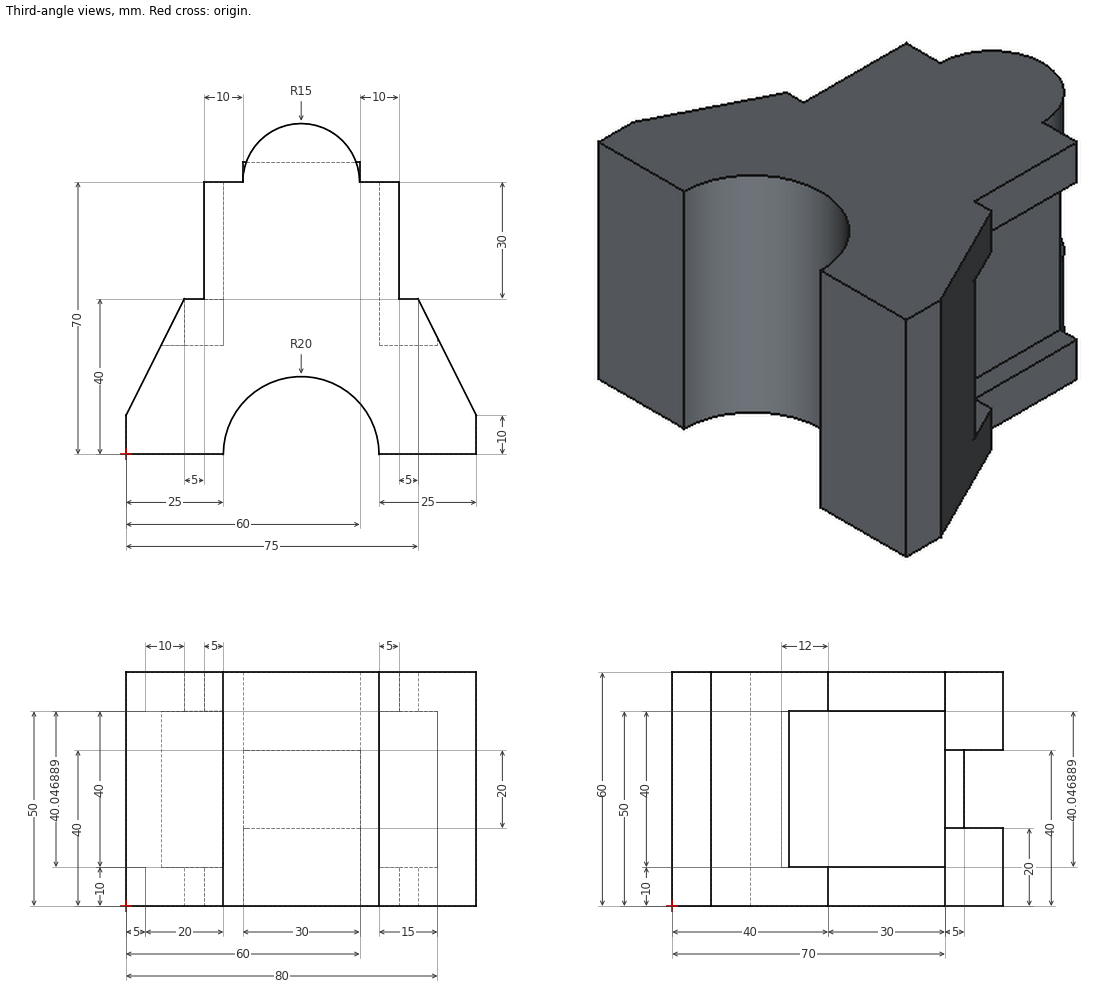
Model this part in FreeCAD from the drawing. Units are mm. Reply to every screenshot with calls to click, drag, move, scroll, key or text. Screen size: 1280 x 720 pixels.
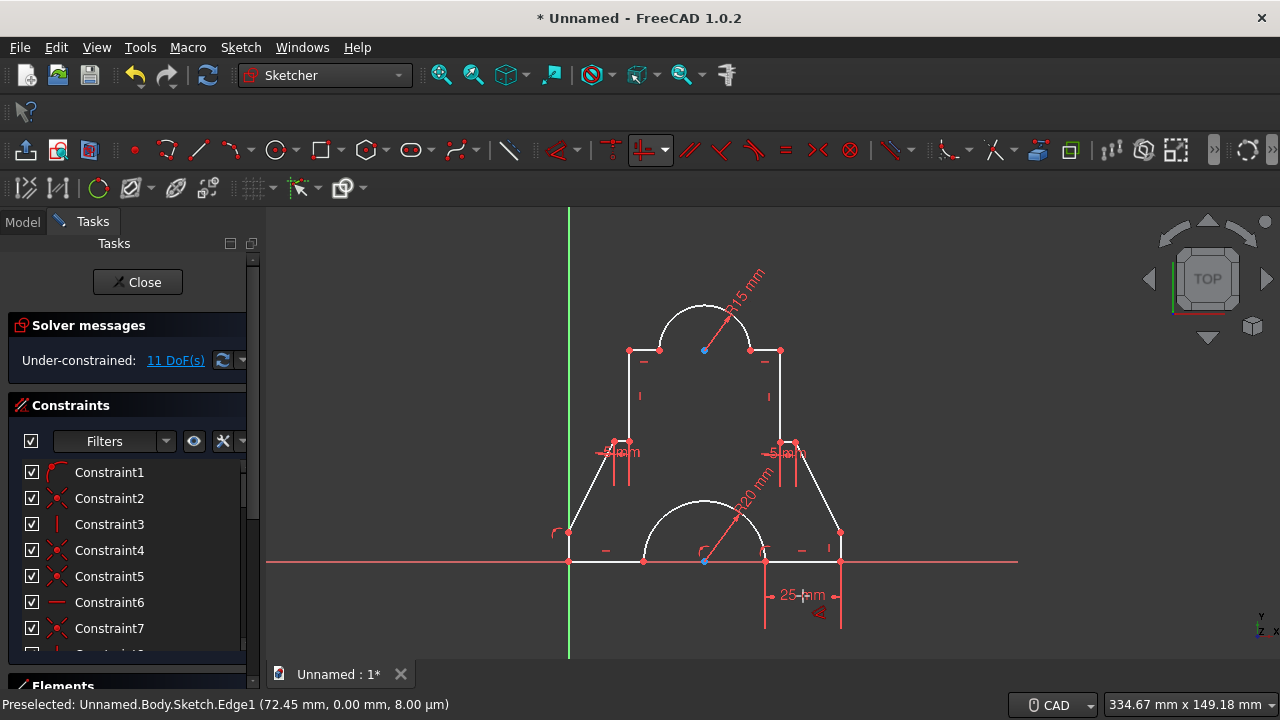
scroll(841, 550, up, 2)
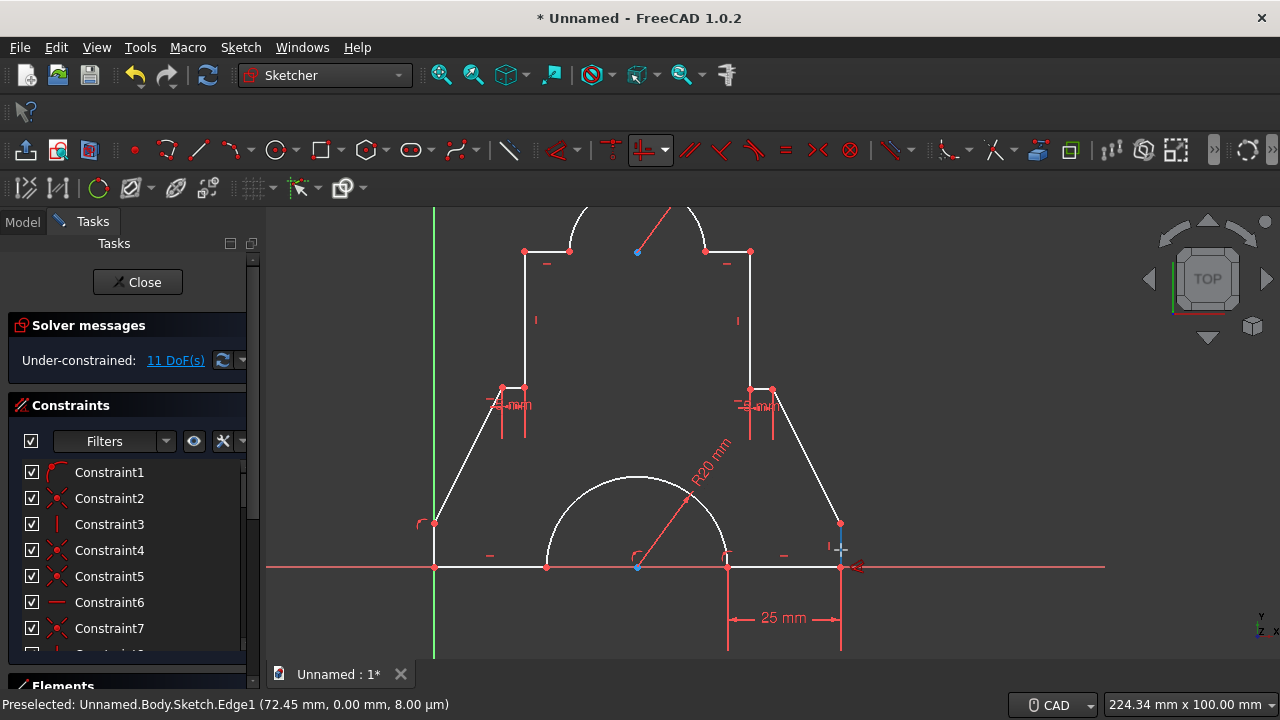
click(841, 550)
click(875, 546)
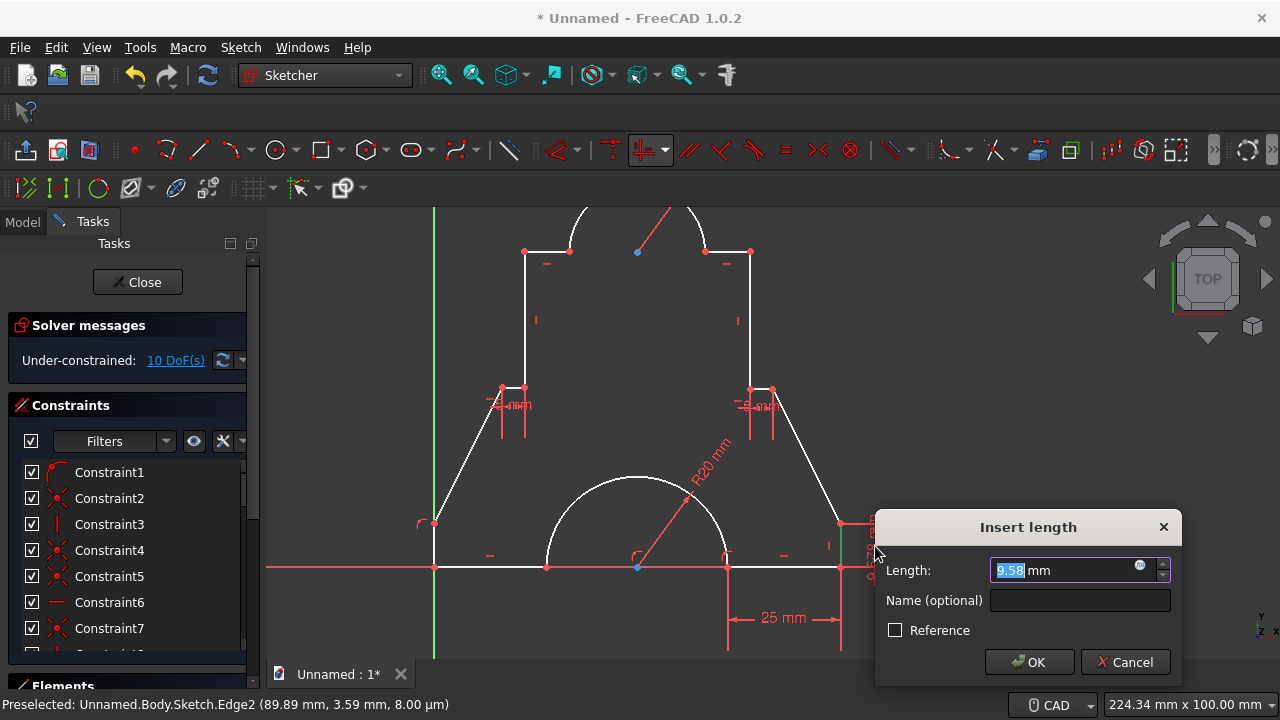
text(10)
key(Return)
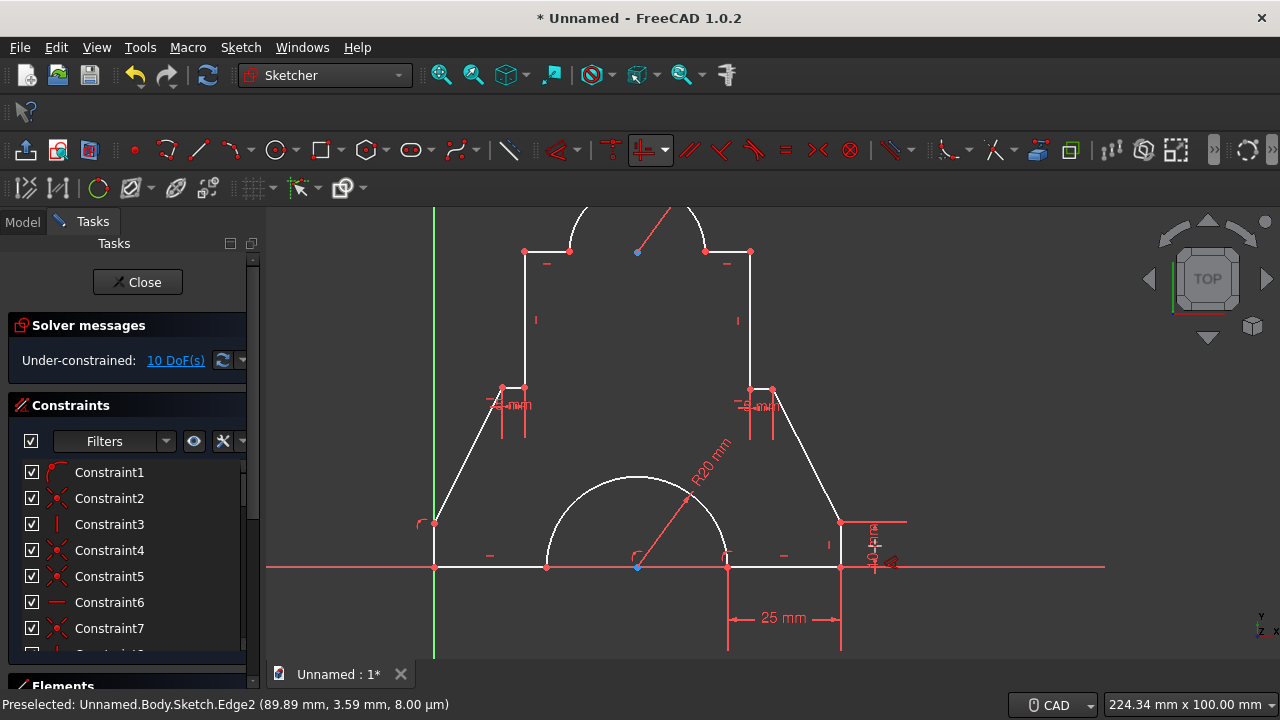
click(750, 348)
click(784, 321)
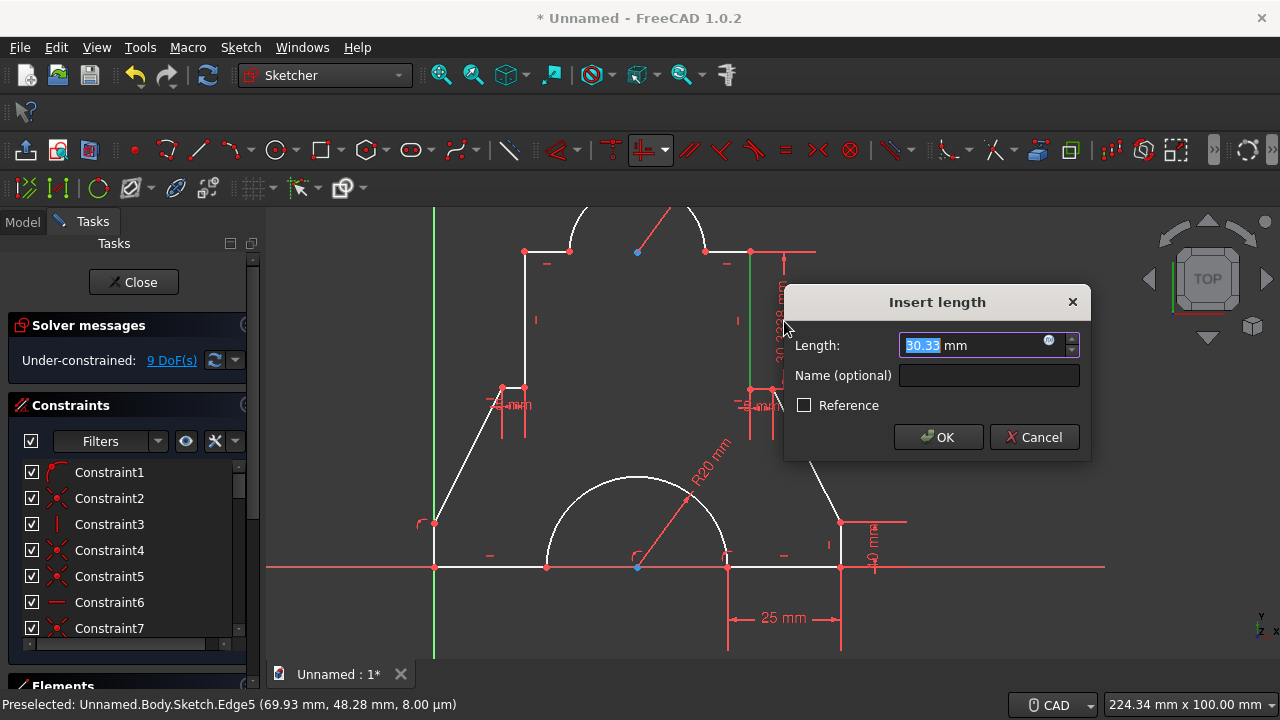
text(30)
key(Return)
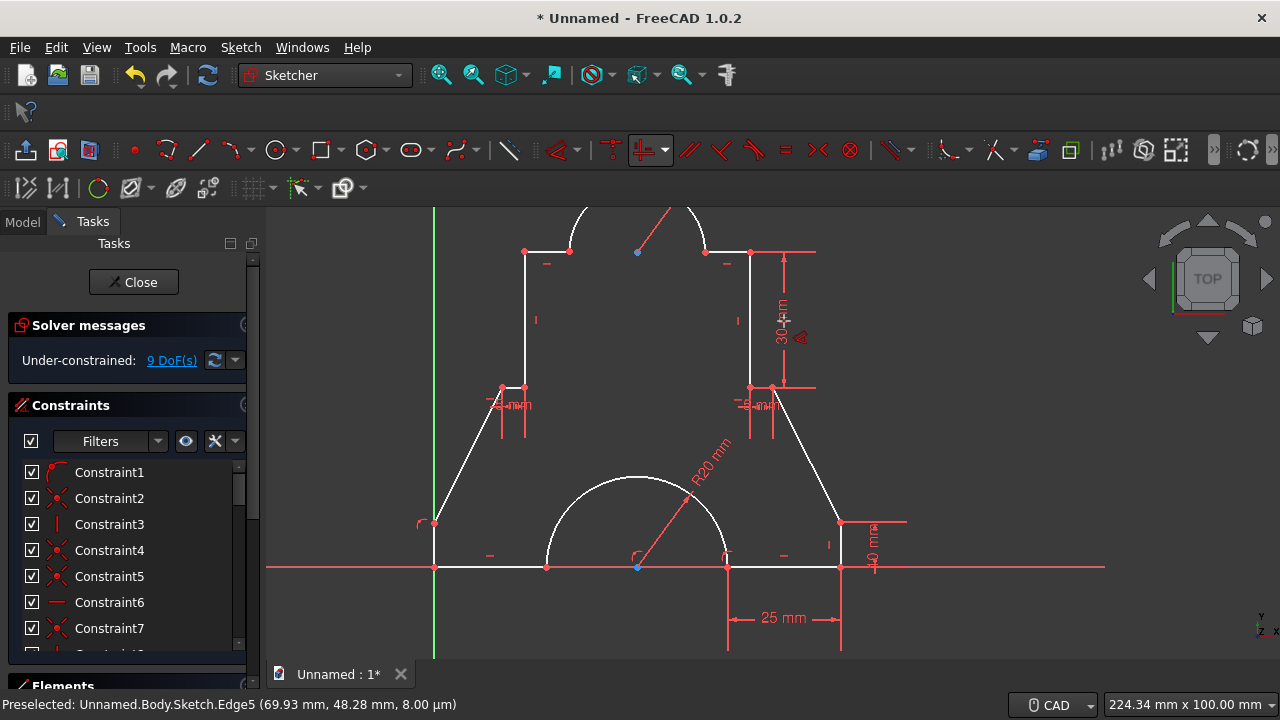
click(737, 252)
click(728, 286)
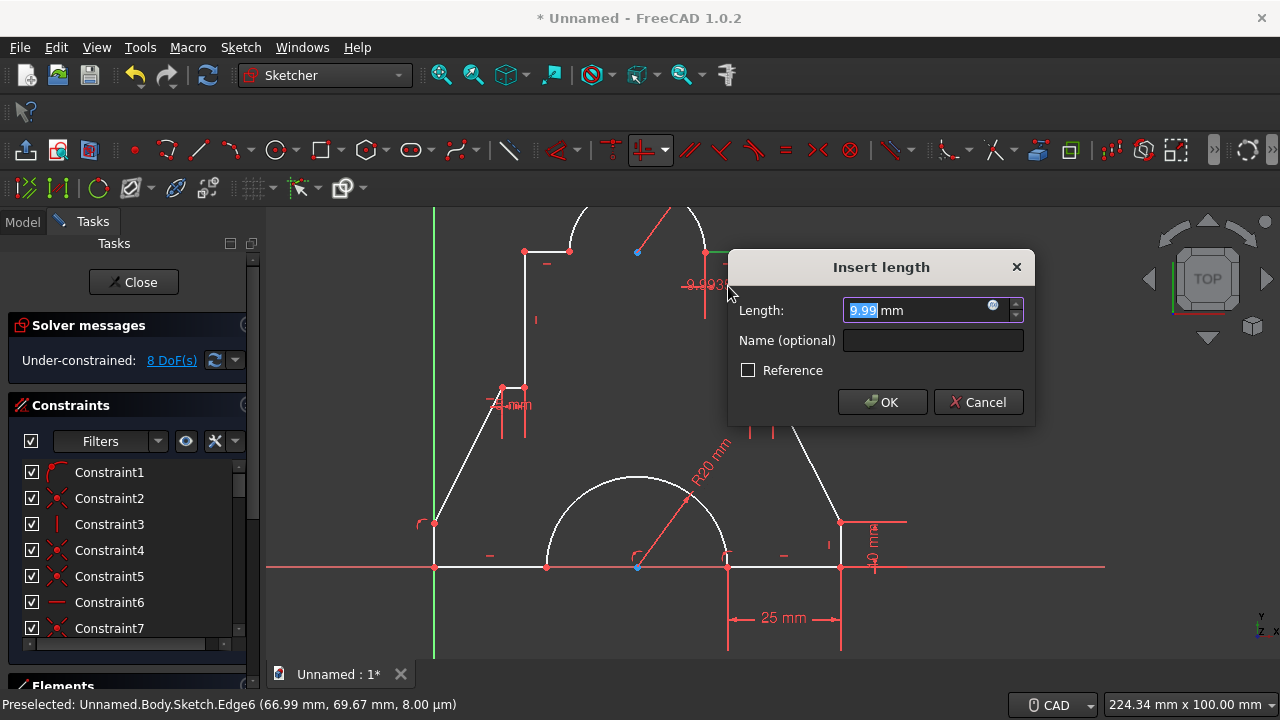
text(10)
key(Return)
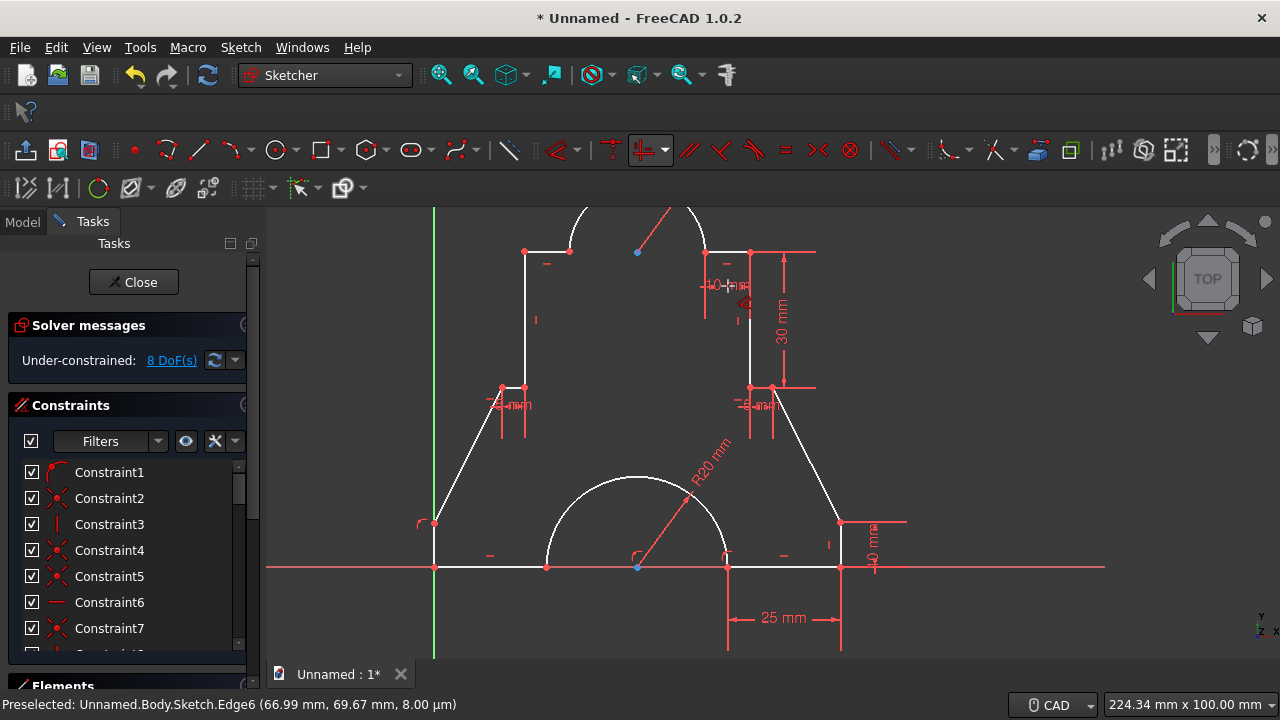
click(556, 252)
click(547, 286)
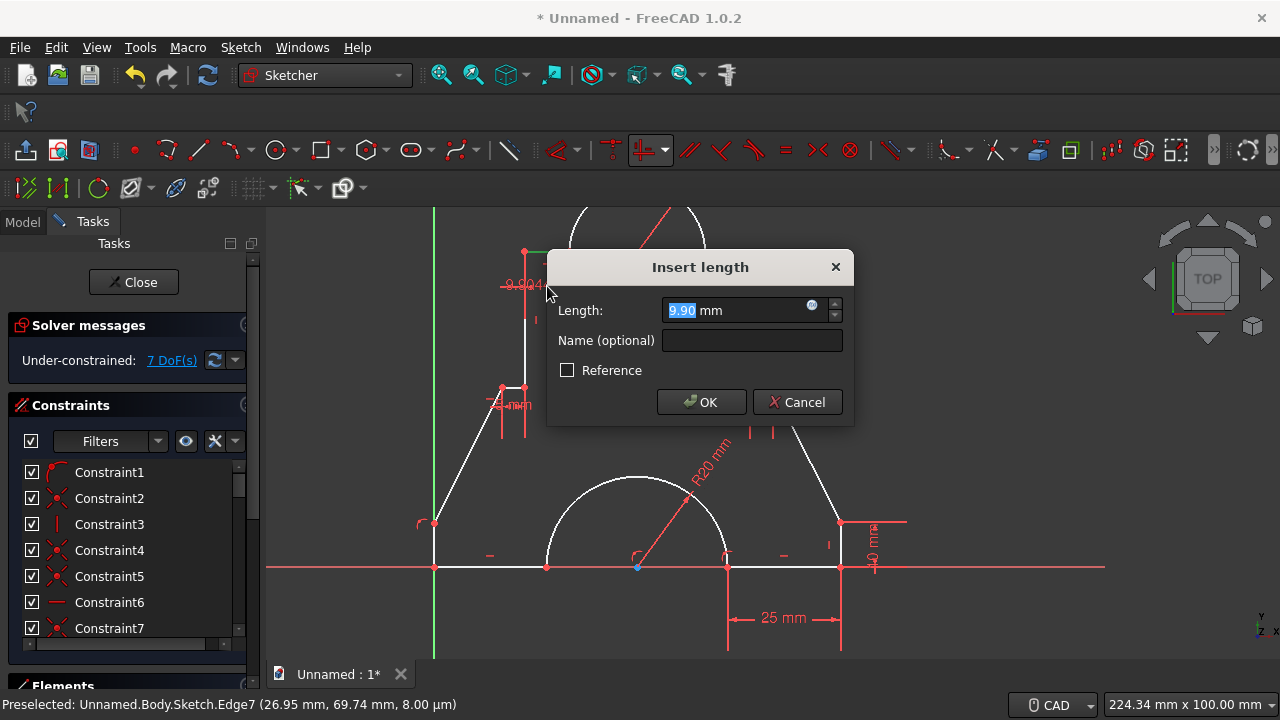
text(10)
key(Return)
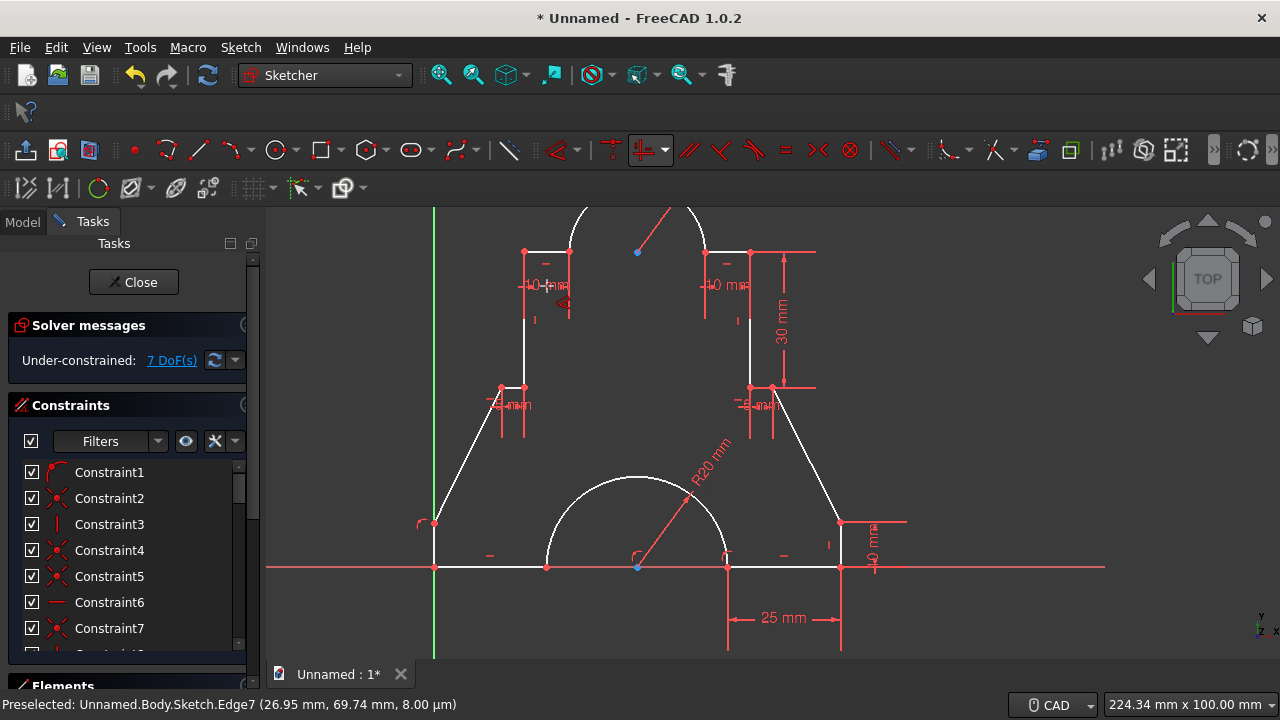
click(524, 293)
click(490, 320)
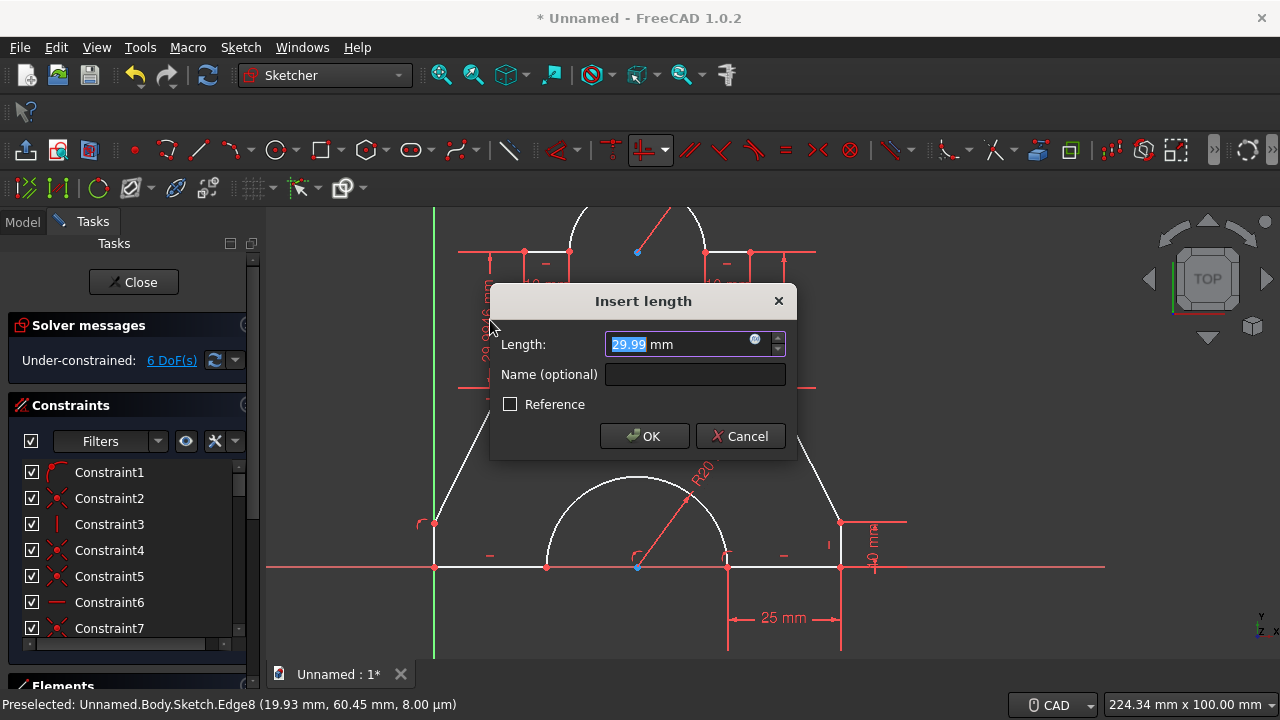
text(30)
key(Return)